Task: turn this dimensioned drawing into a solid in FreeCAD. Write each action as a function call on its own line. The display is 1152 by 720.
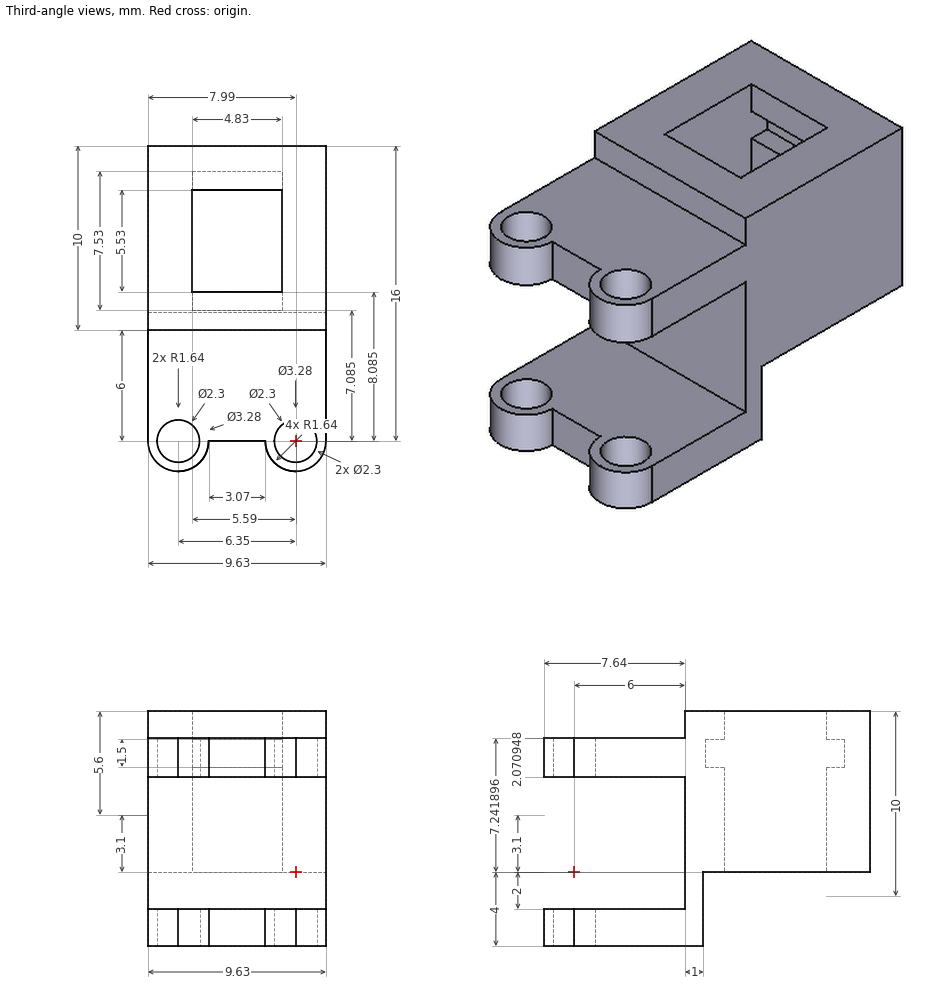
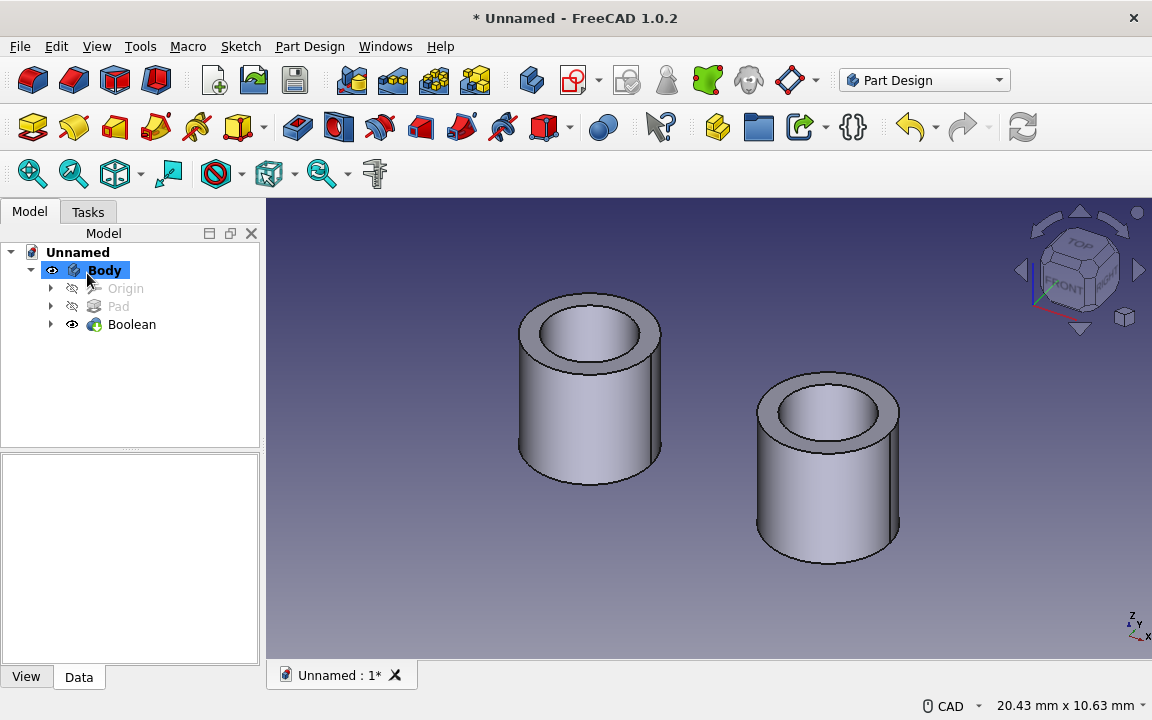
click(572, 80)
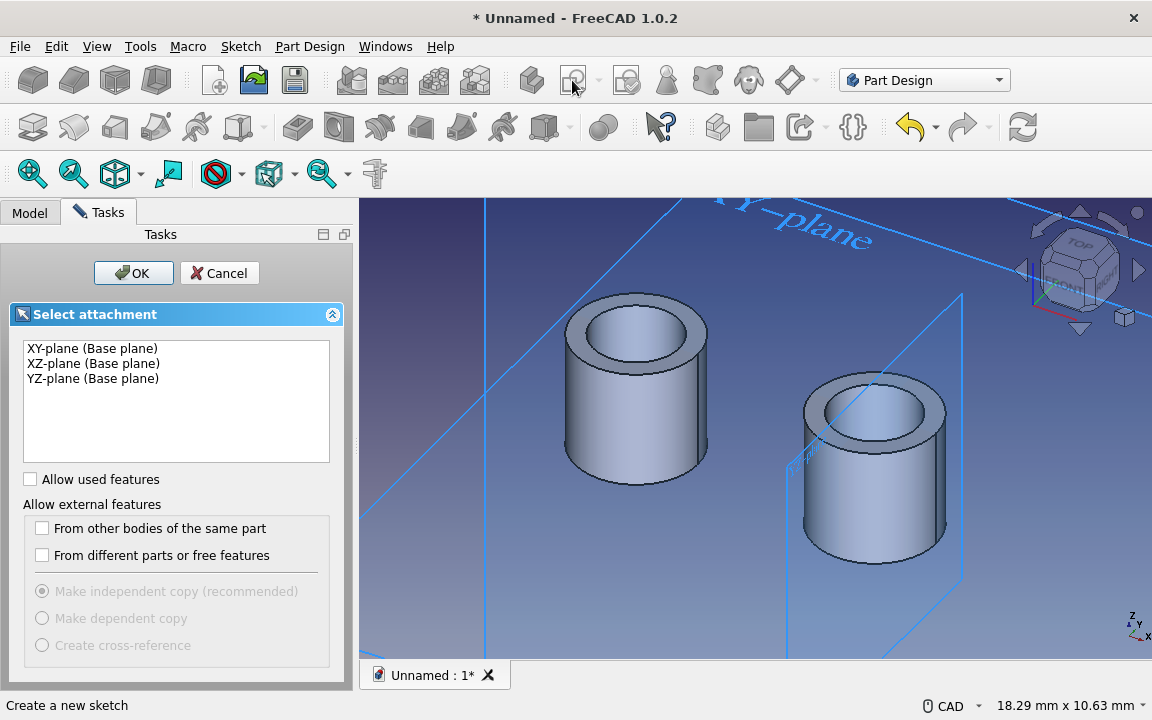
click(84, 348)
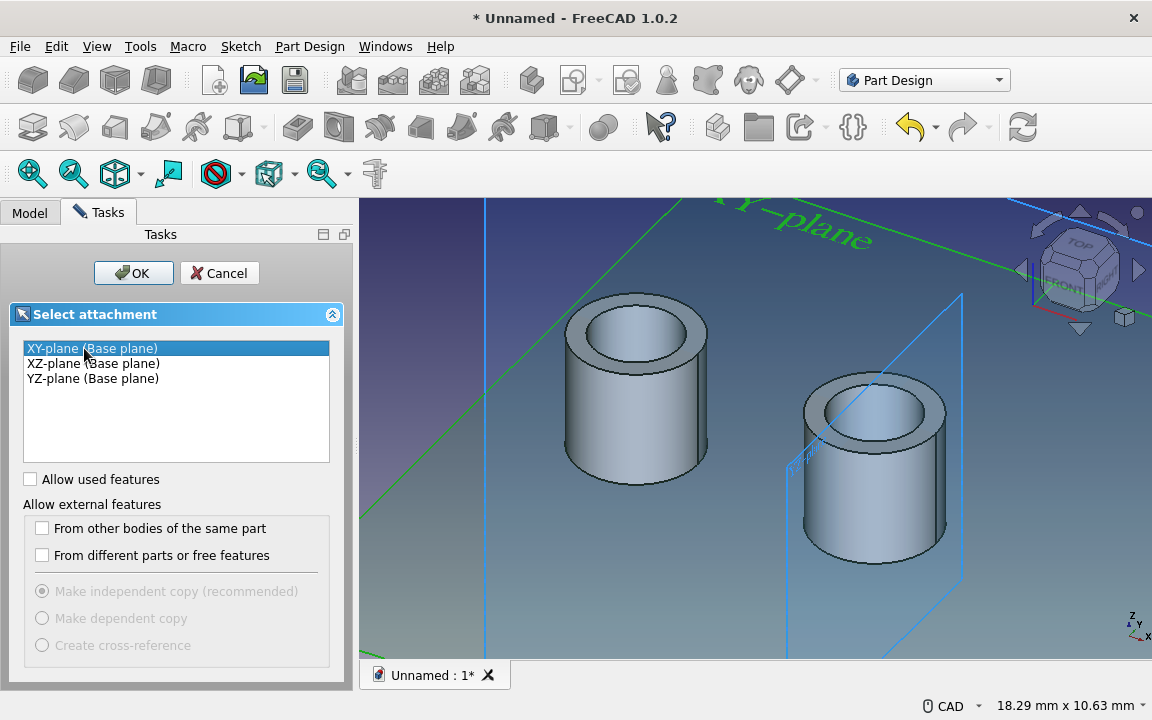
click(134, 273)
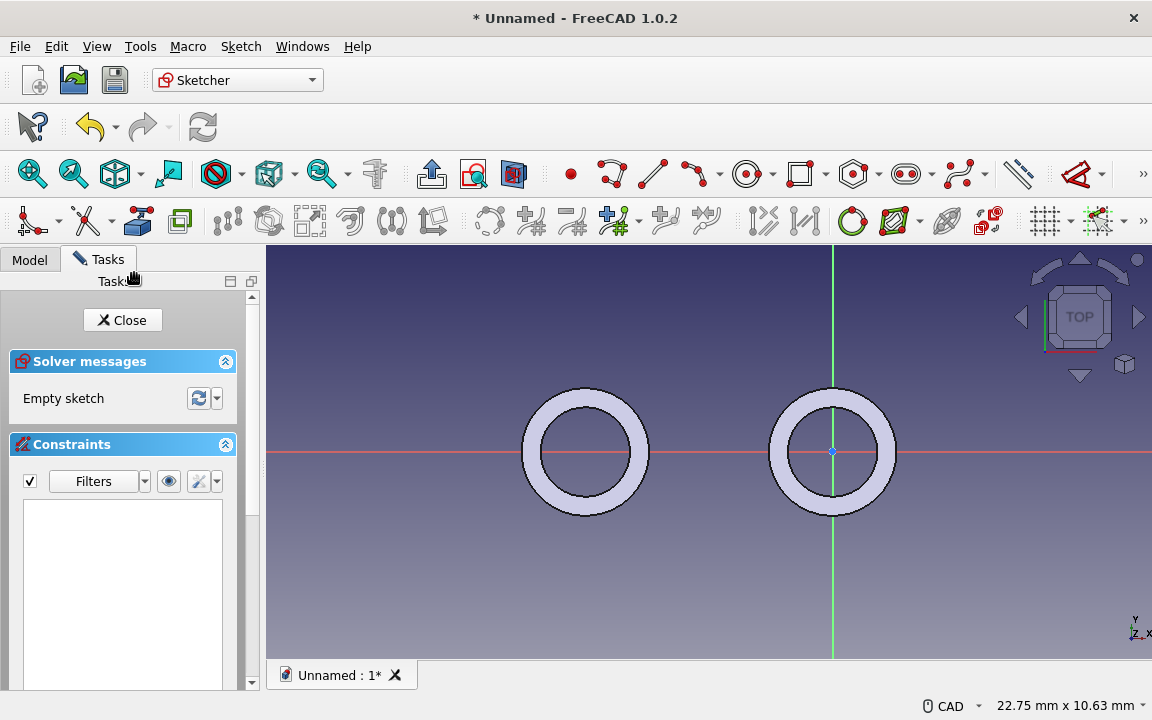
click(514, 174)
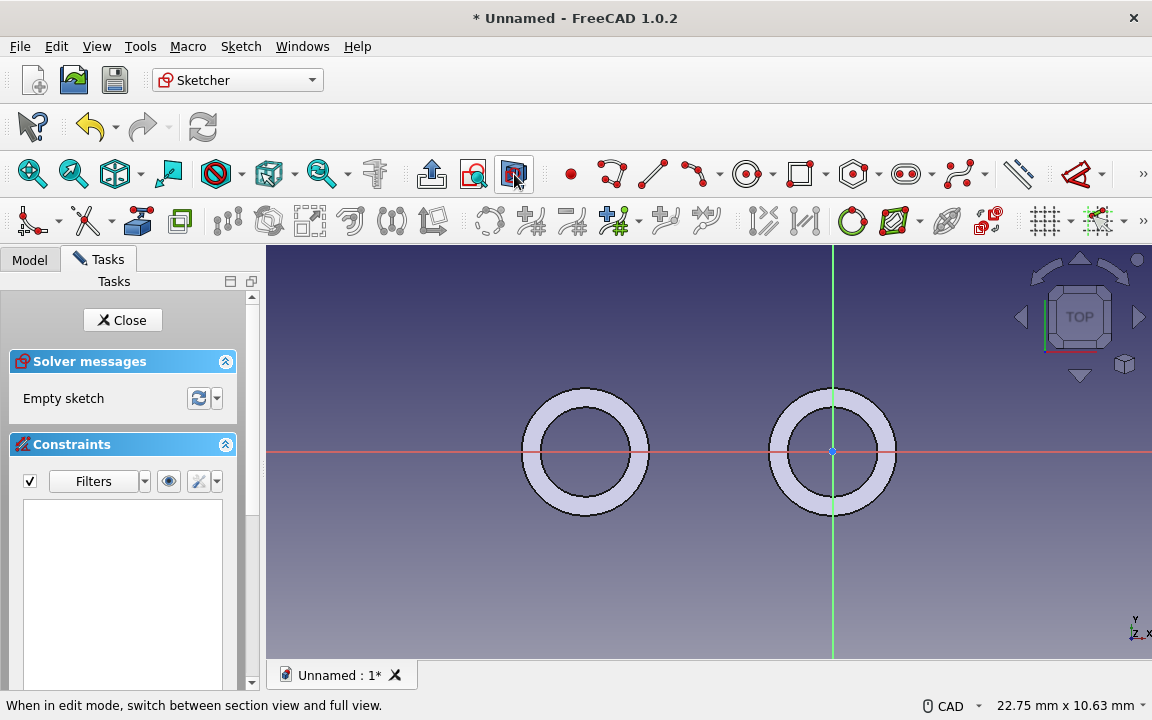
scroll(601, 631, down, 5)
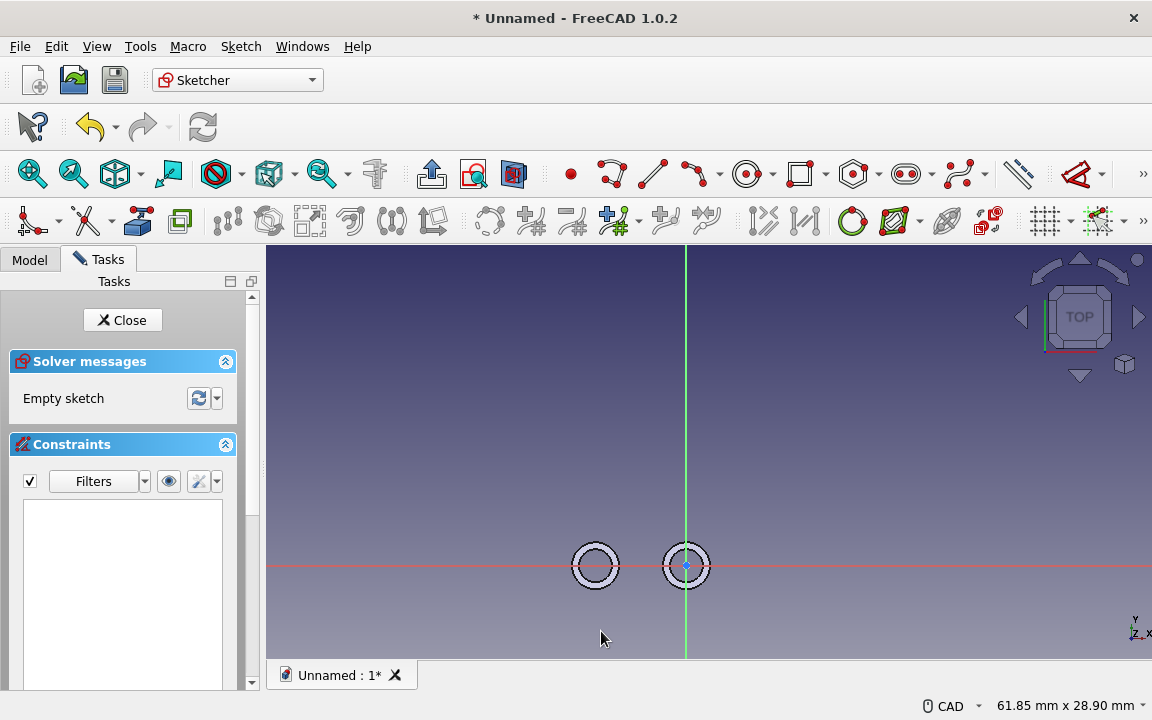
click(653, 174)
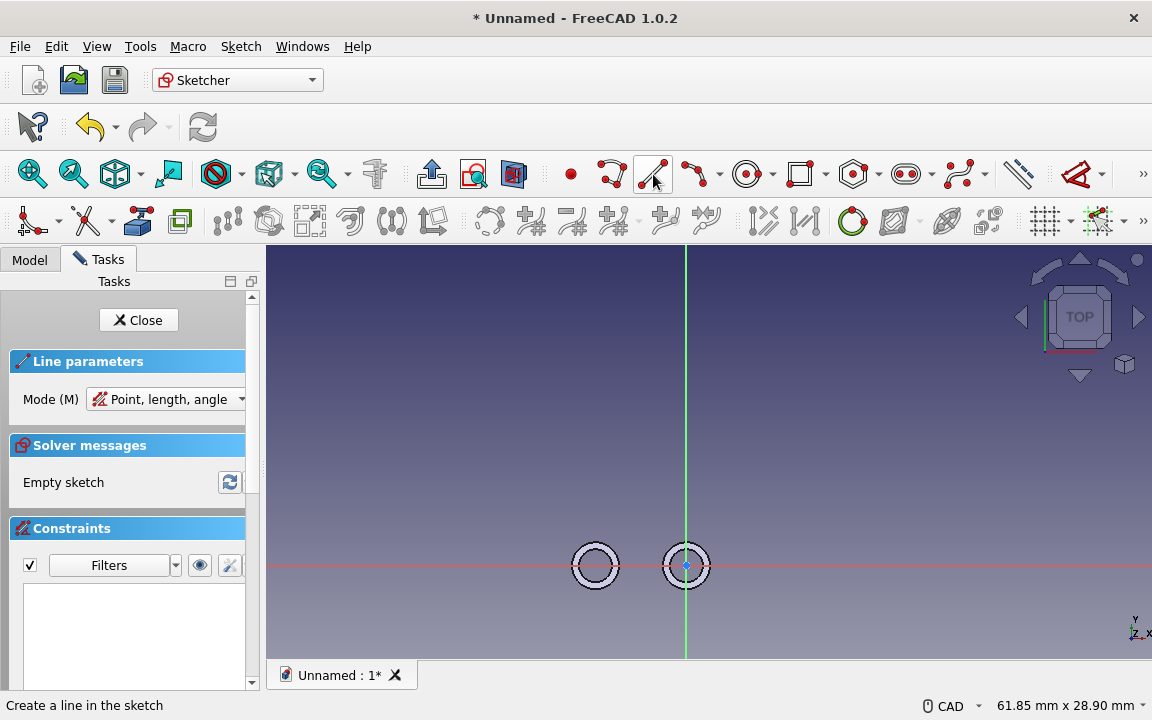
click(619, 566)
click(663, 557)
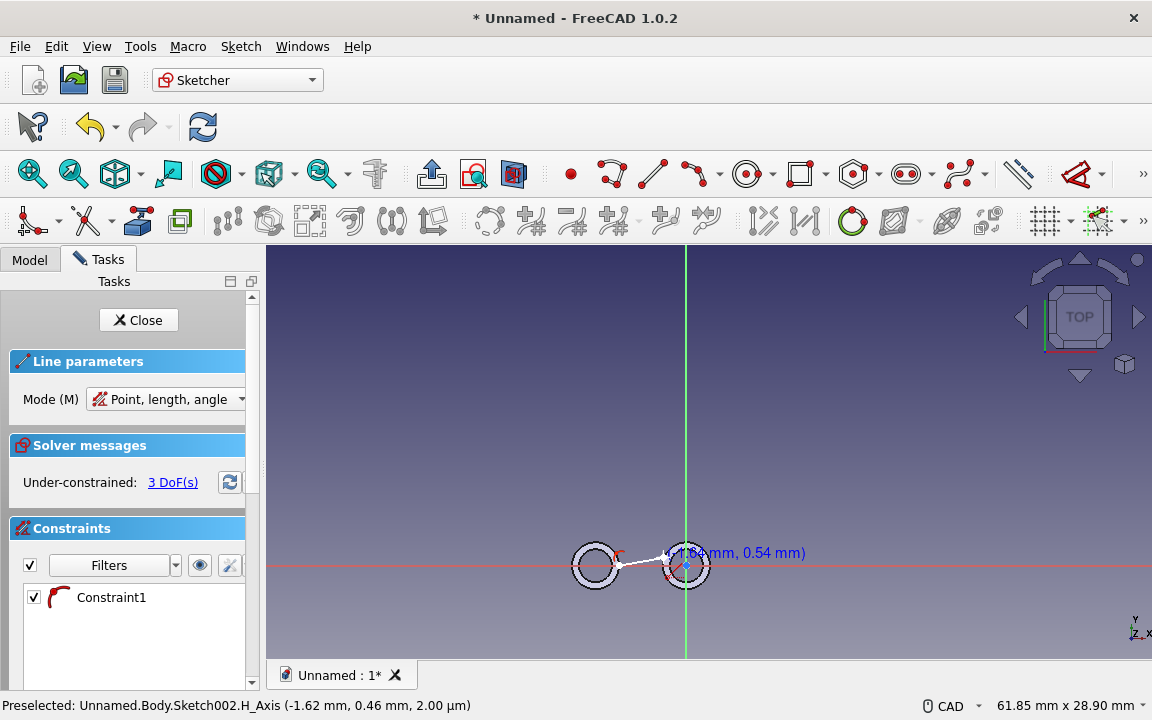
key(g)
key(m)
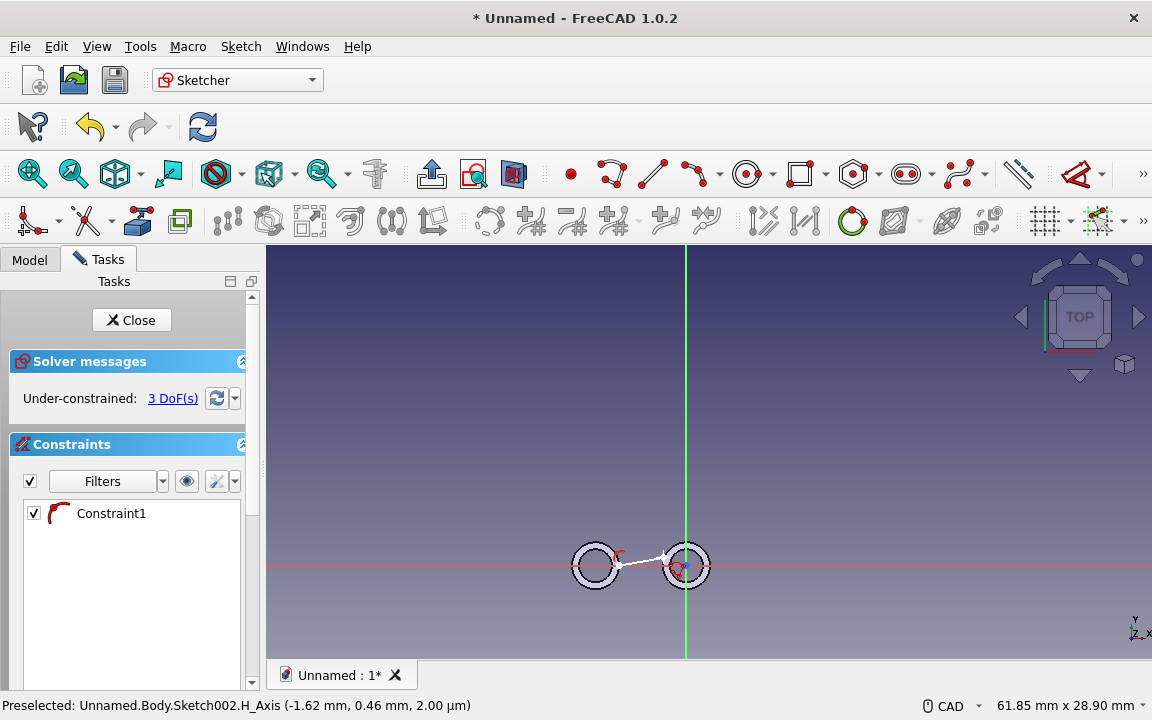
click(710, 566)
click(710, 337)
click(572, 337)
click(572, 566)
right_click(572, 566)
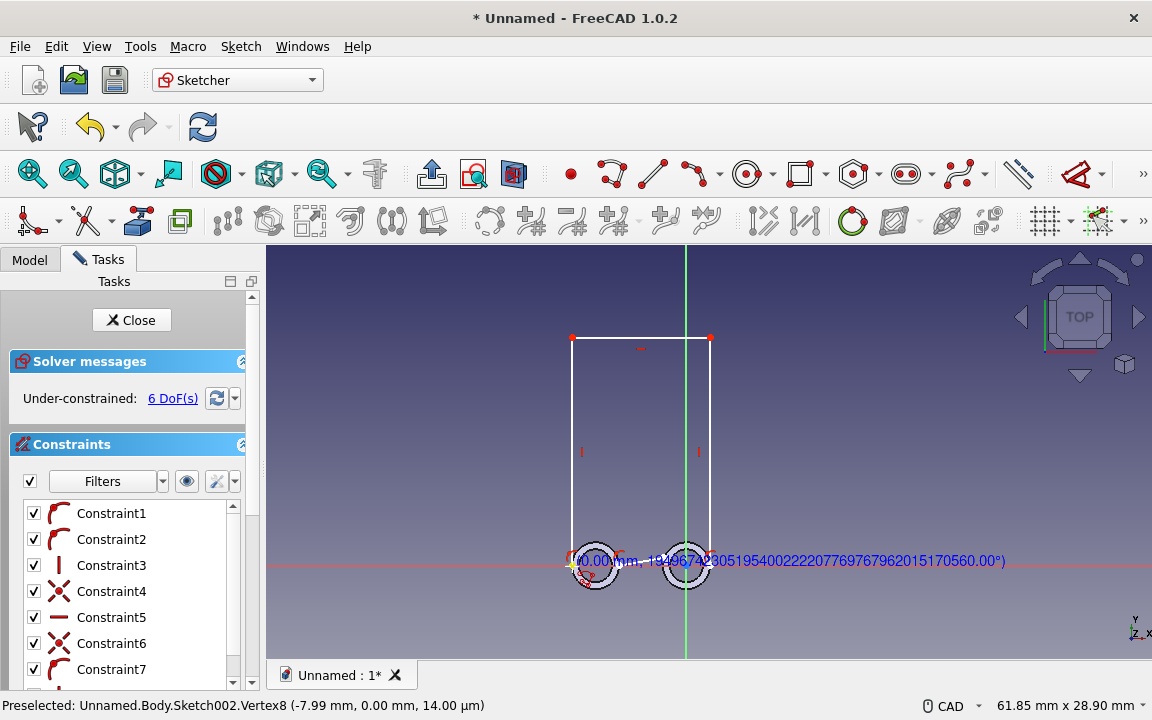
click(694, 174)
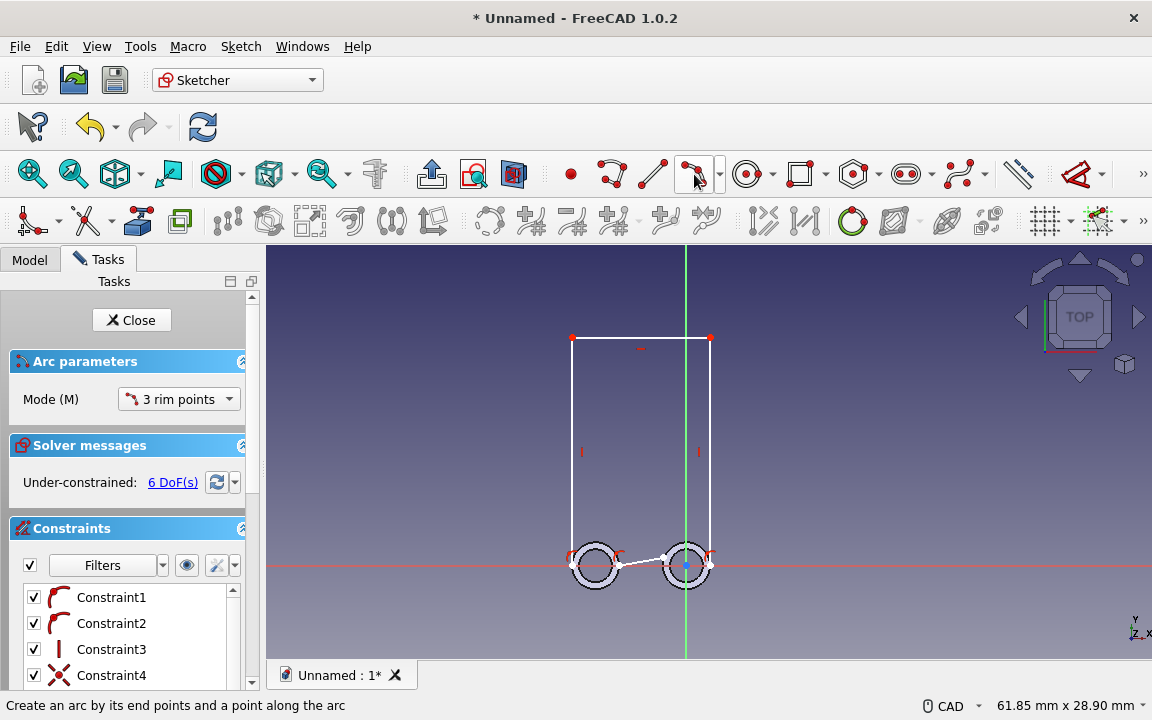
click(663, 558)
click(710, 566)
click(673, 547)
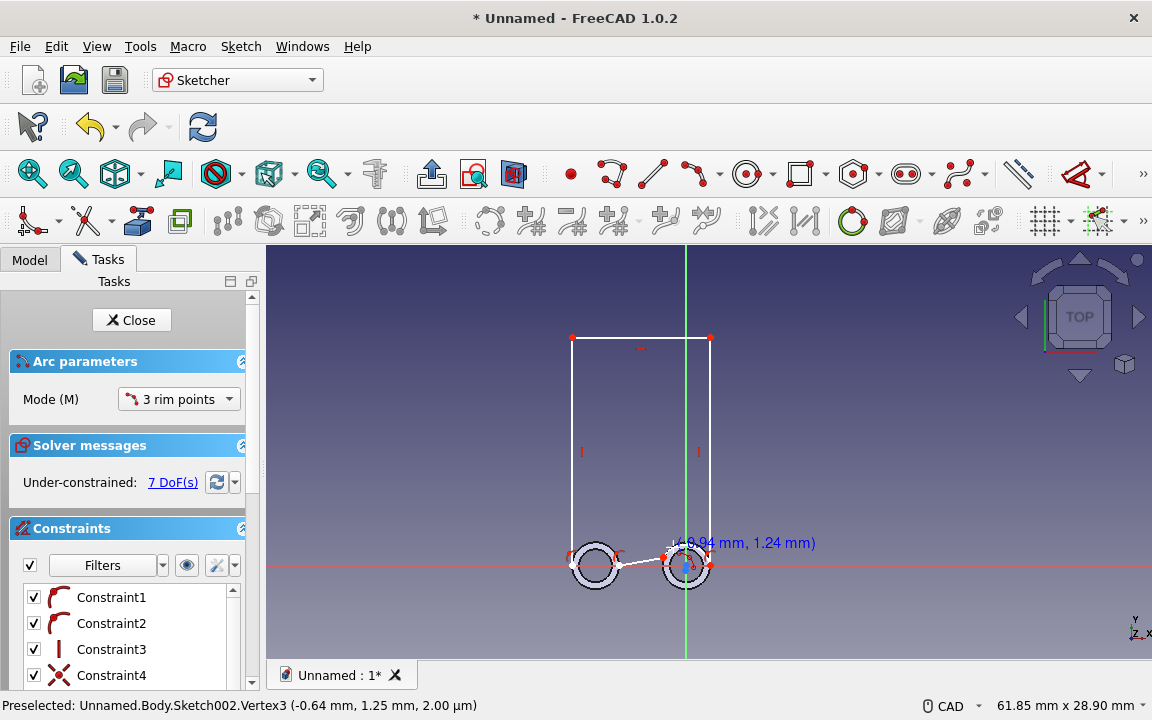
click(572, 566)
click(619, 566)
click(595, 542)
key(Escape)